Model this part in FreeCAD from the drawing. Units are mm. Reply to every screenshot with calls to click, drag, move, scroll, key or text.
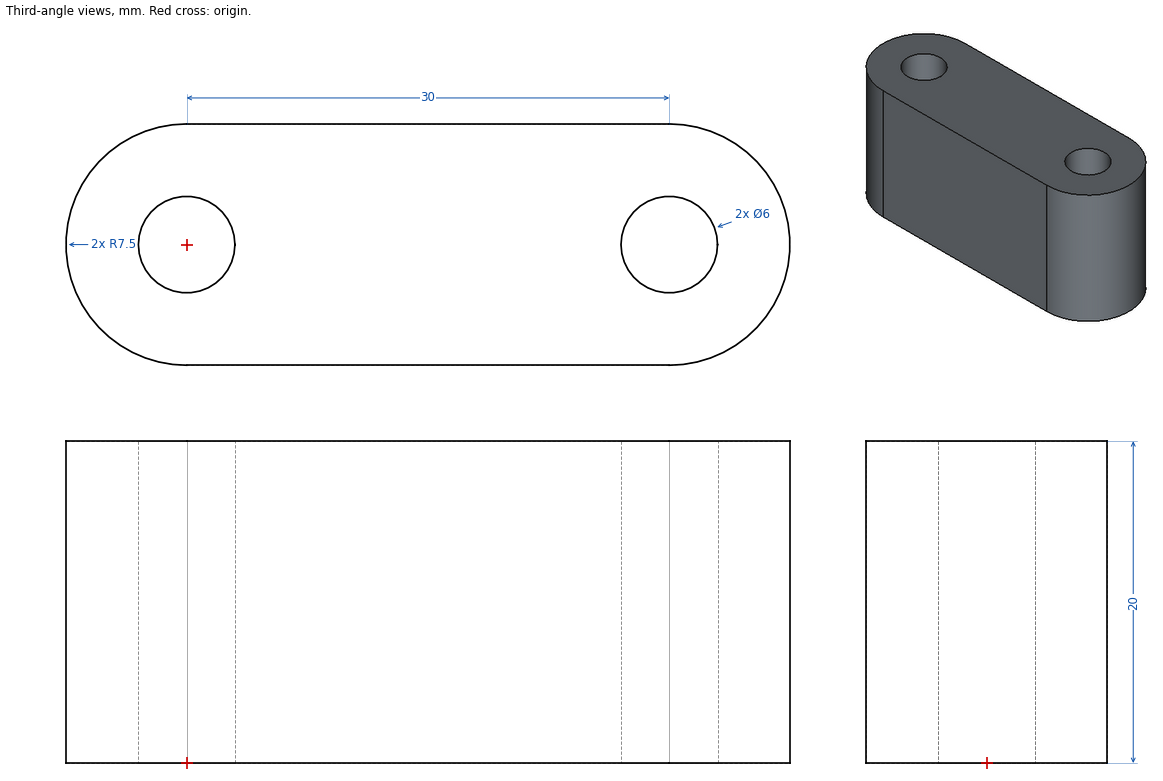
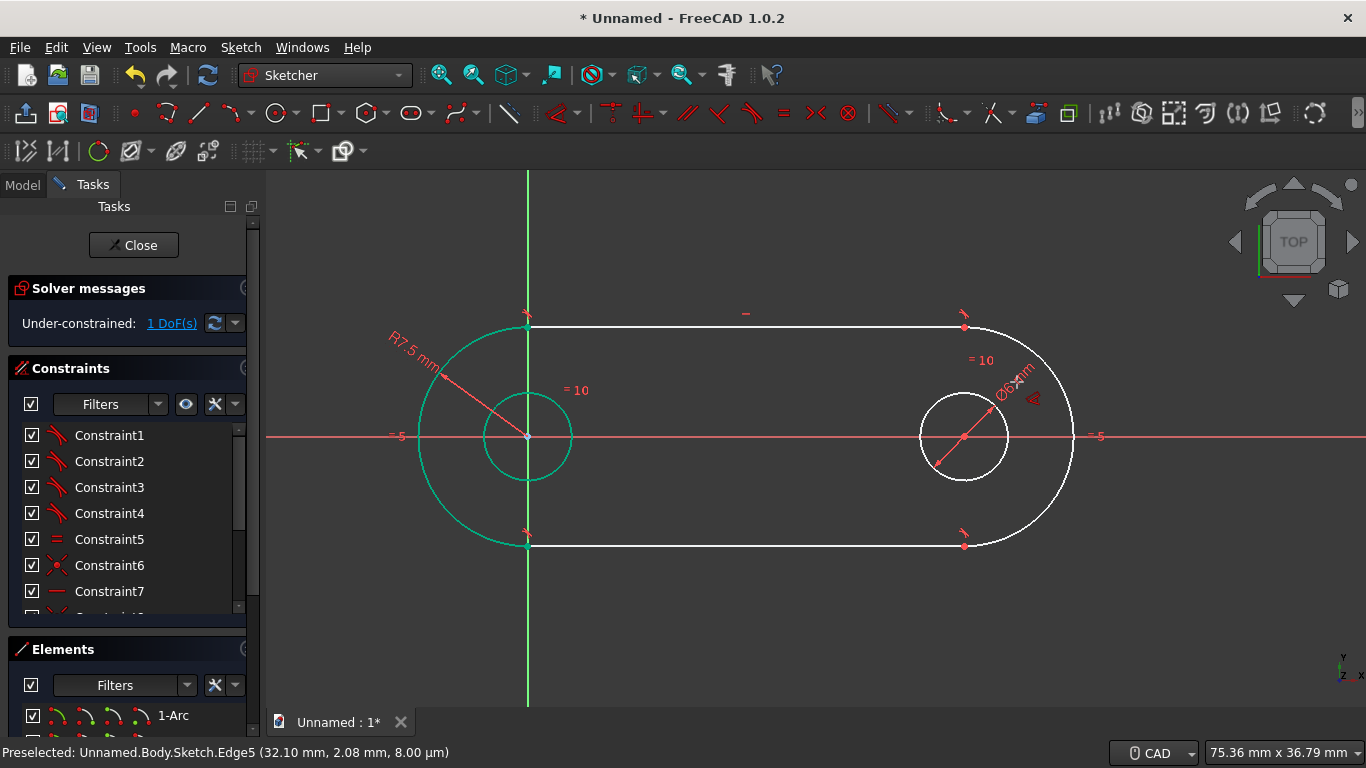
click(659, 327)
click(746, 293)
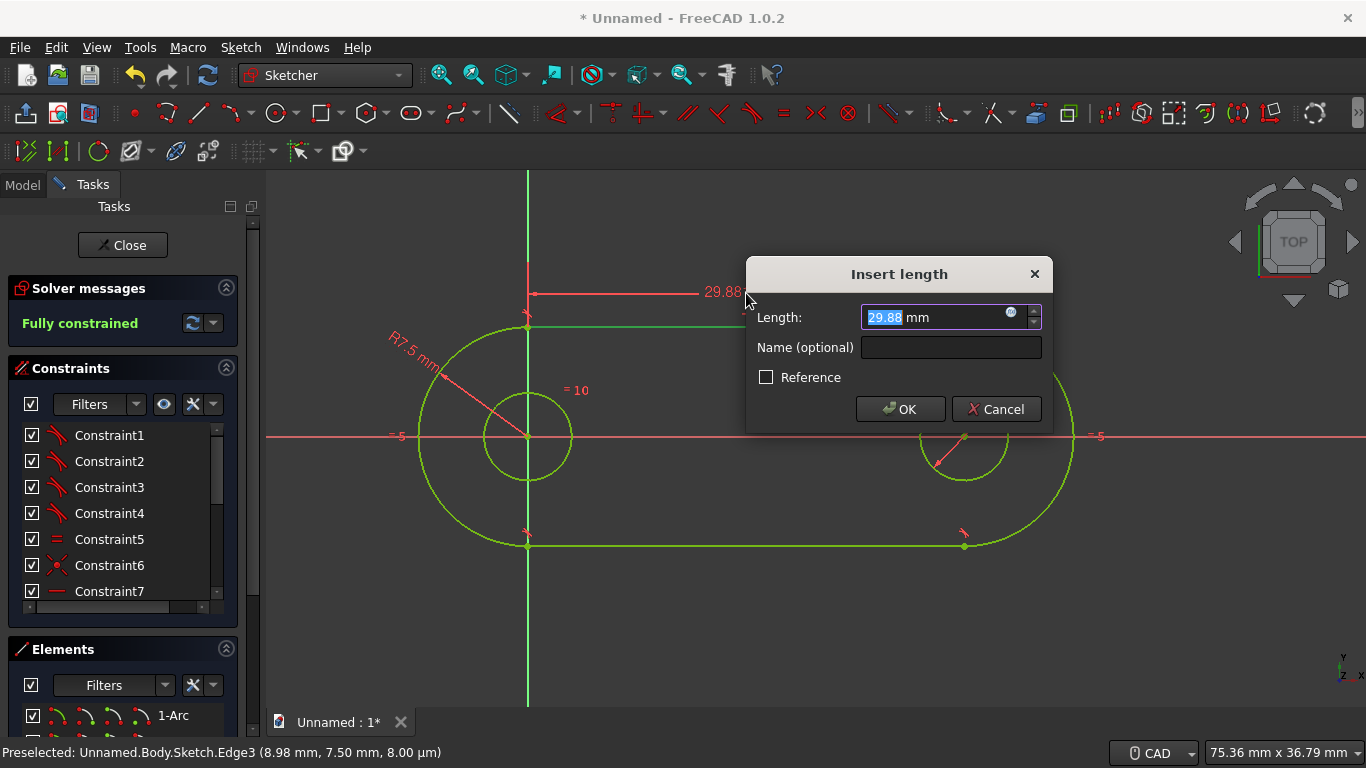
text(30)
key(Return)
key(Escape)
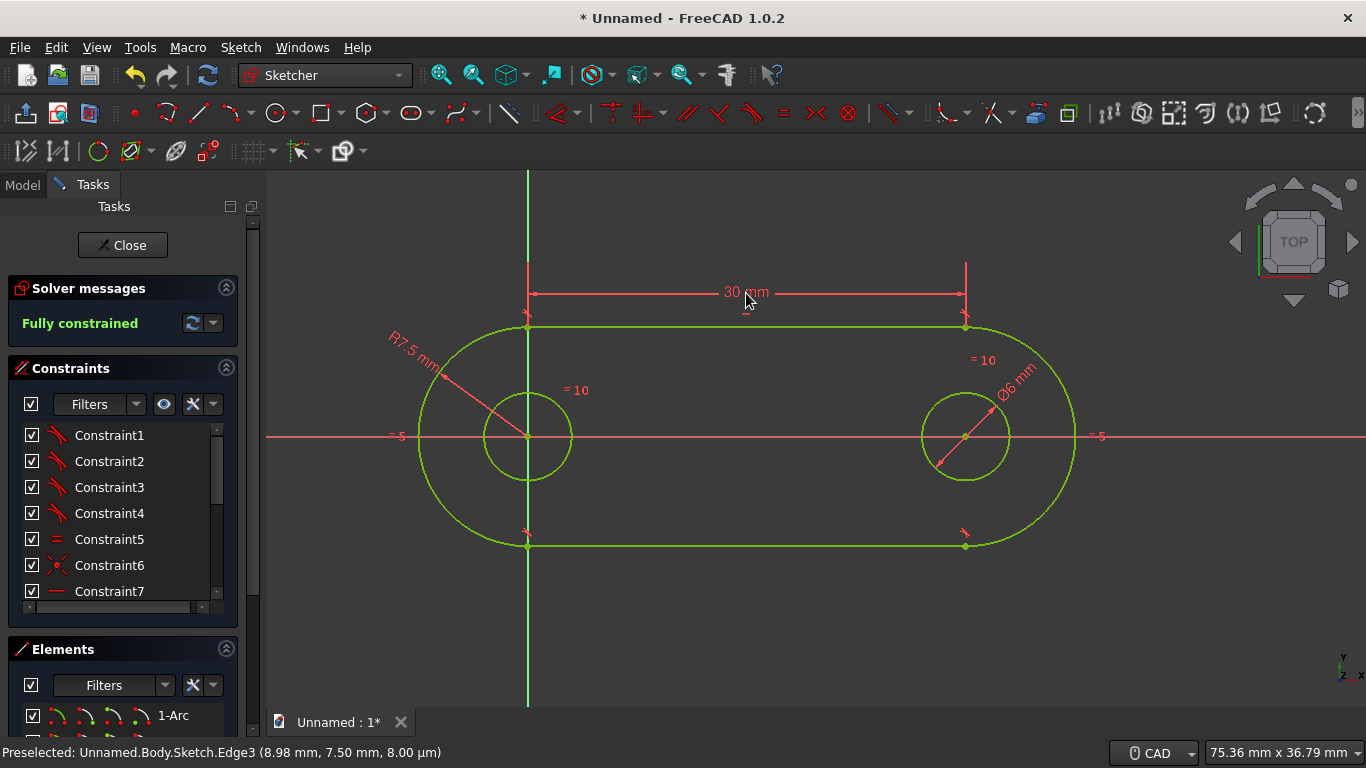
click(123, 245)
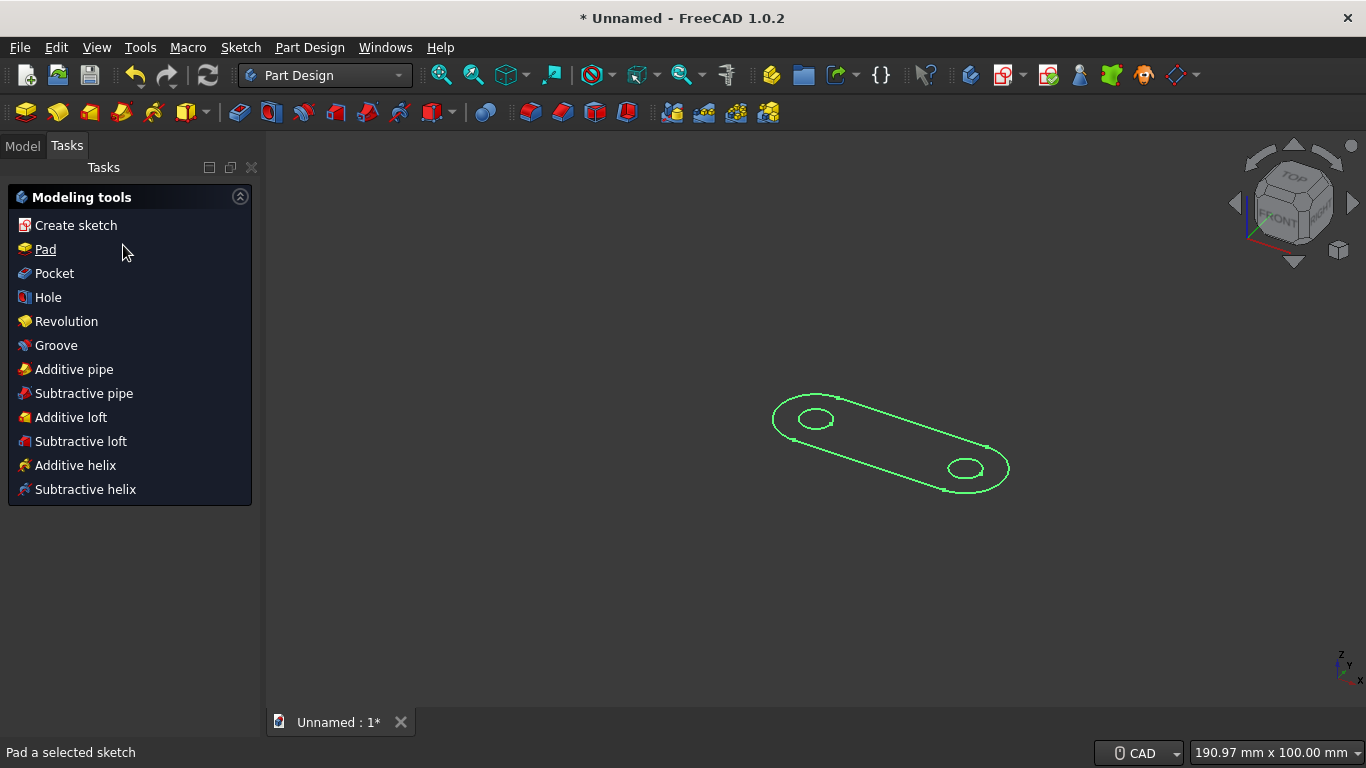
click(26, 112)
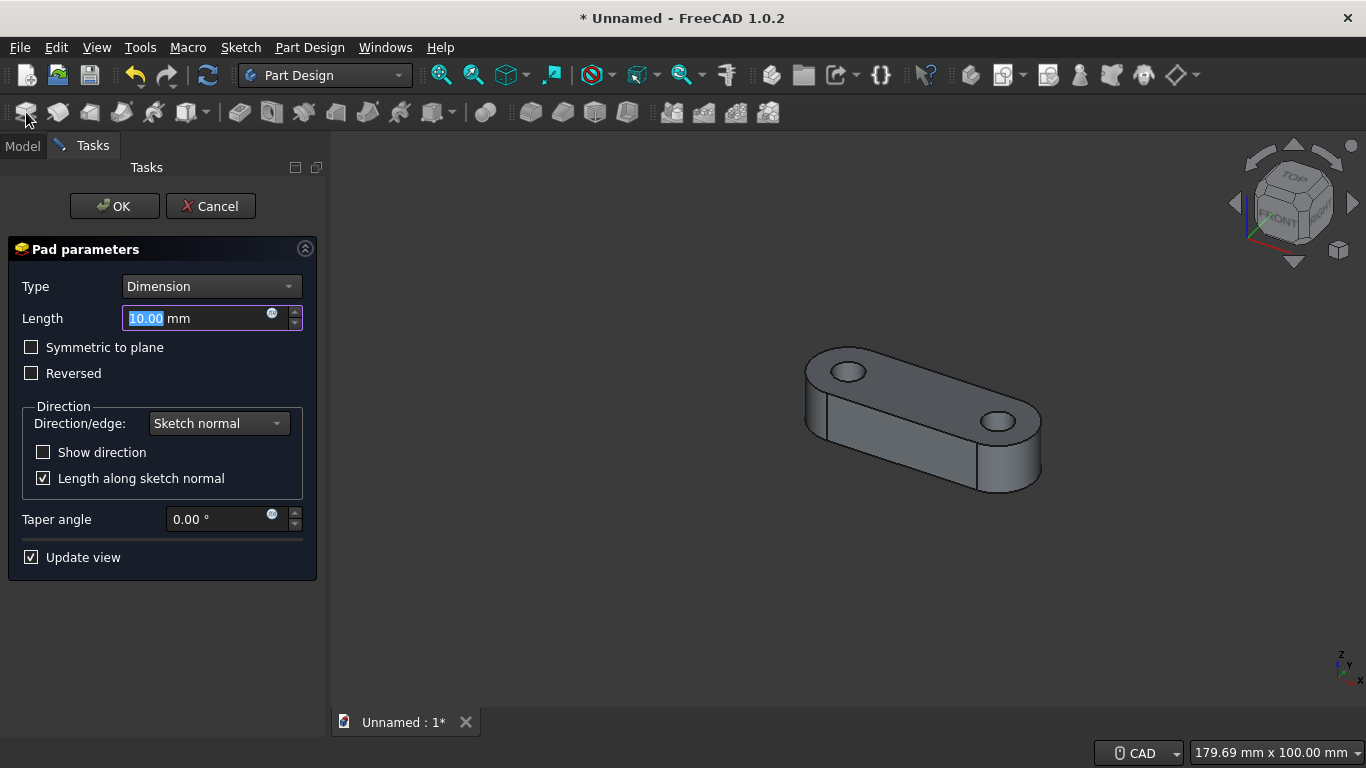
text(20)
key(Tab)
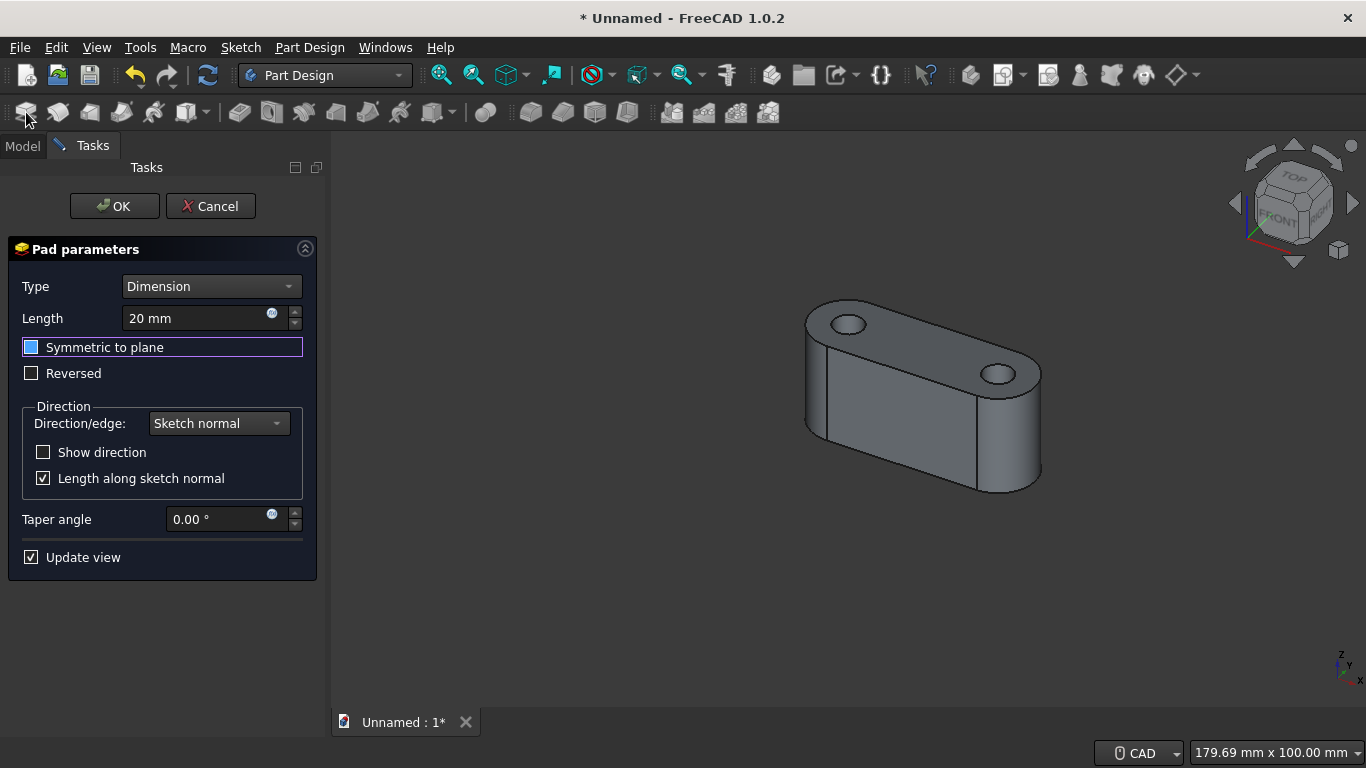
click(115, 206)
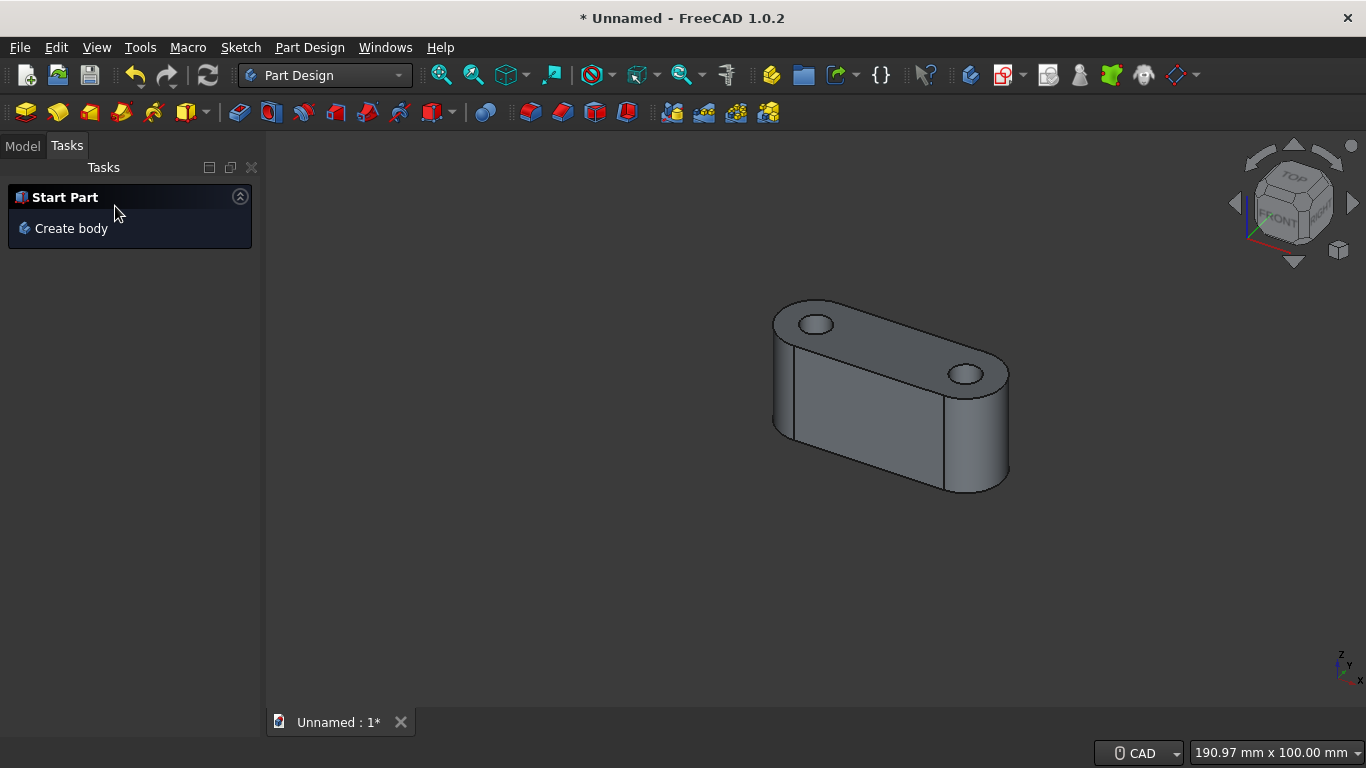
key(0)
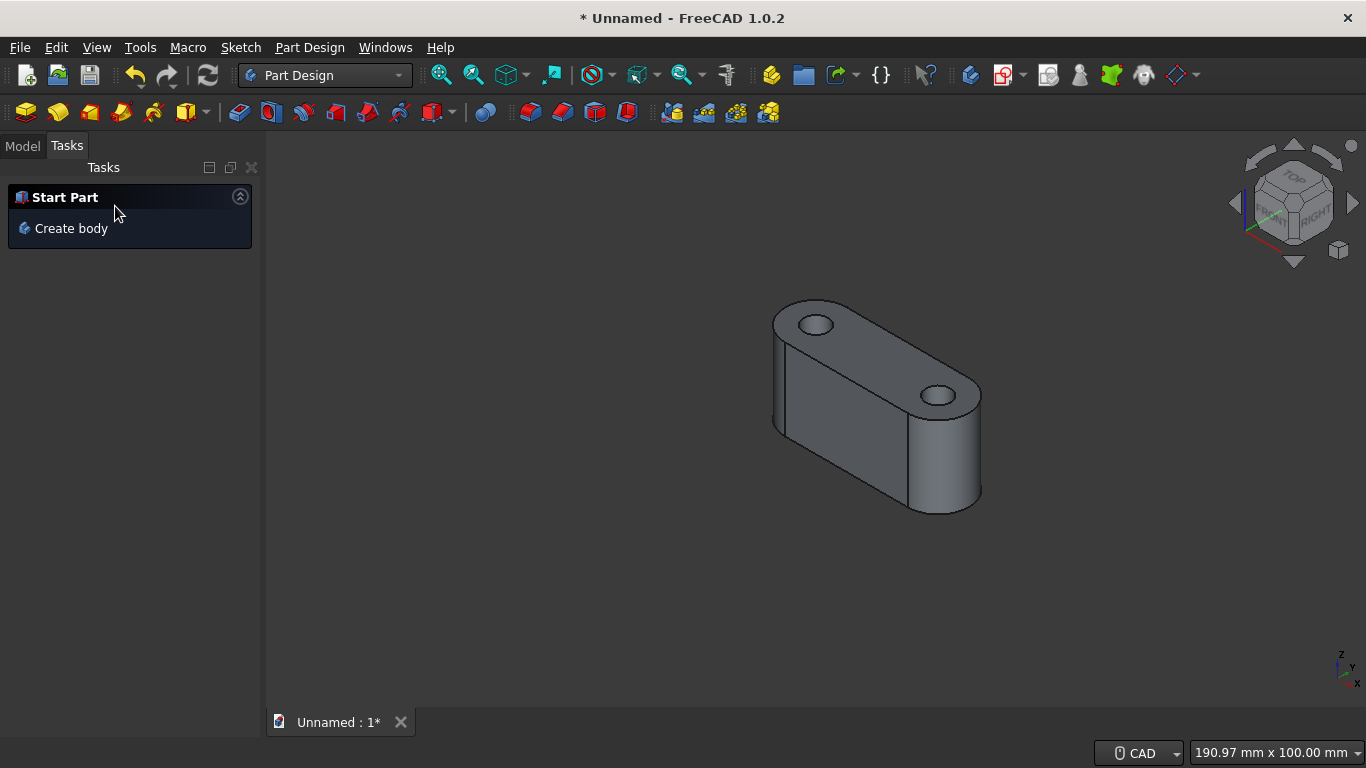
key(v)
key(f)